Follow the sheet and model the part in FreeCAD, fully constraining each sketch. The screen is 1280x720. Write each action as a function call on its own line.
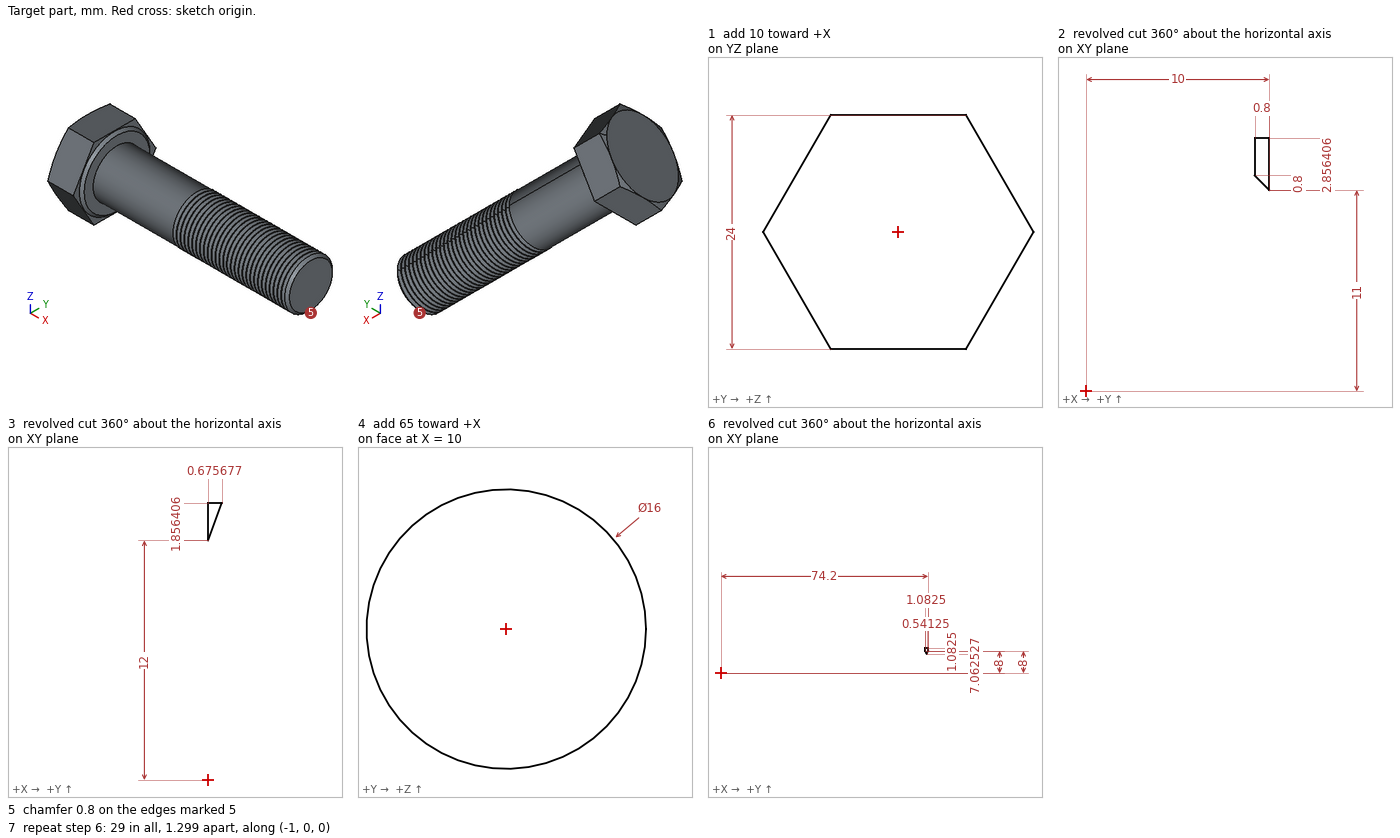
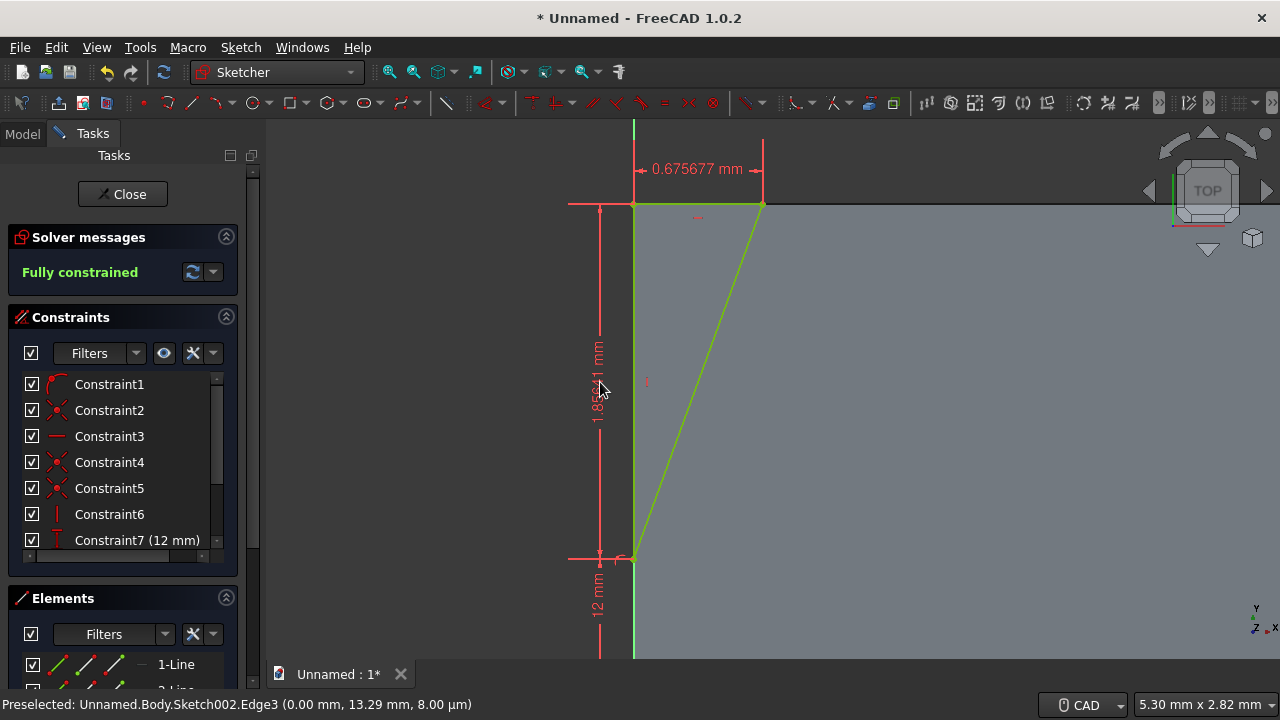
click(123, 194)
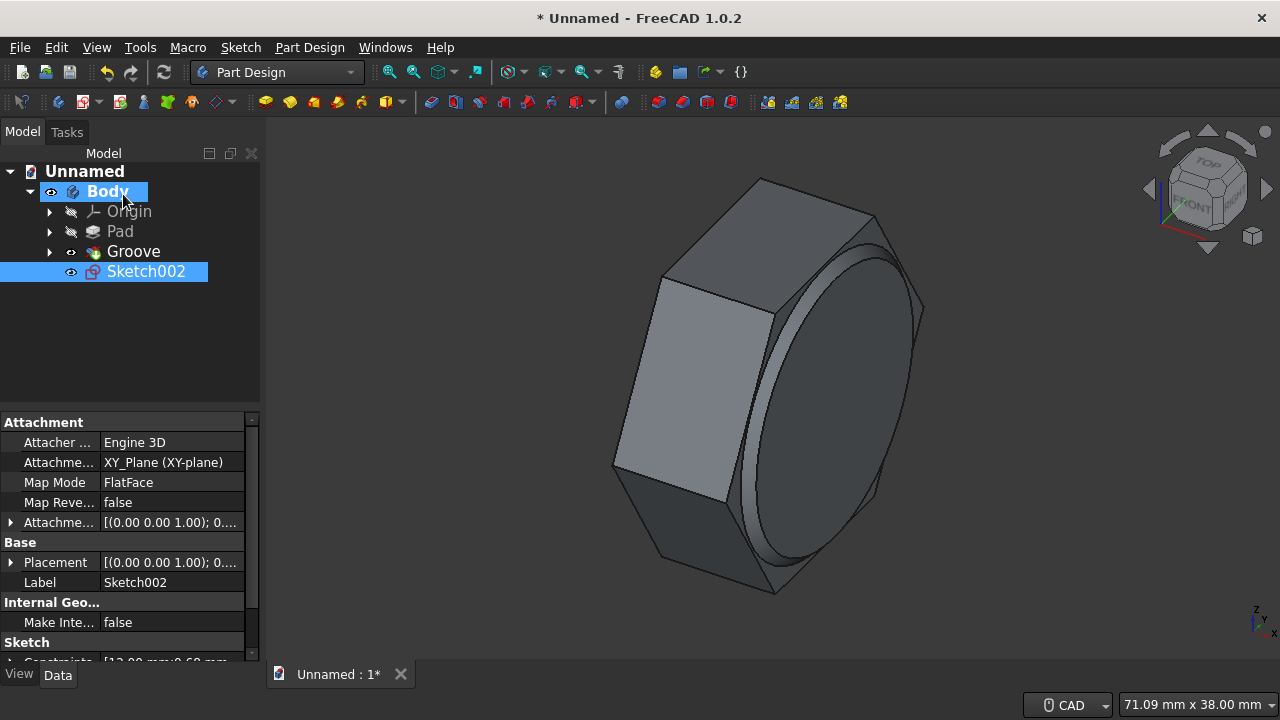
click(480, 102)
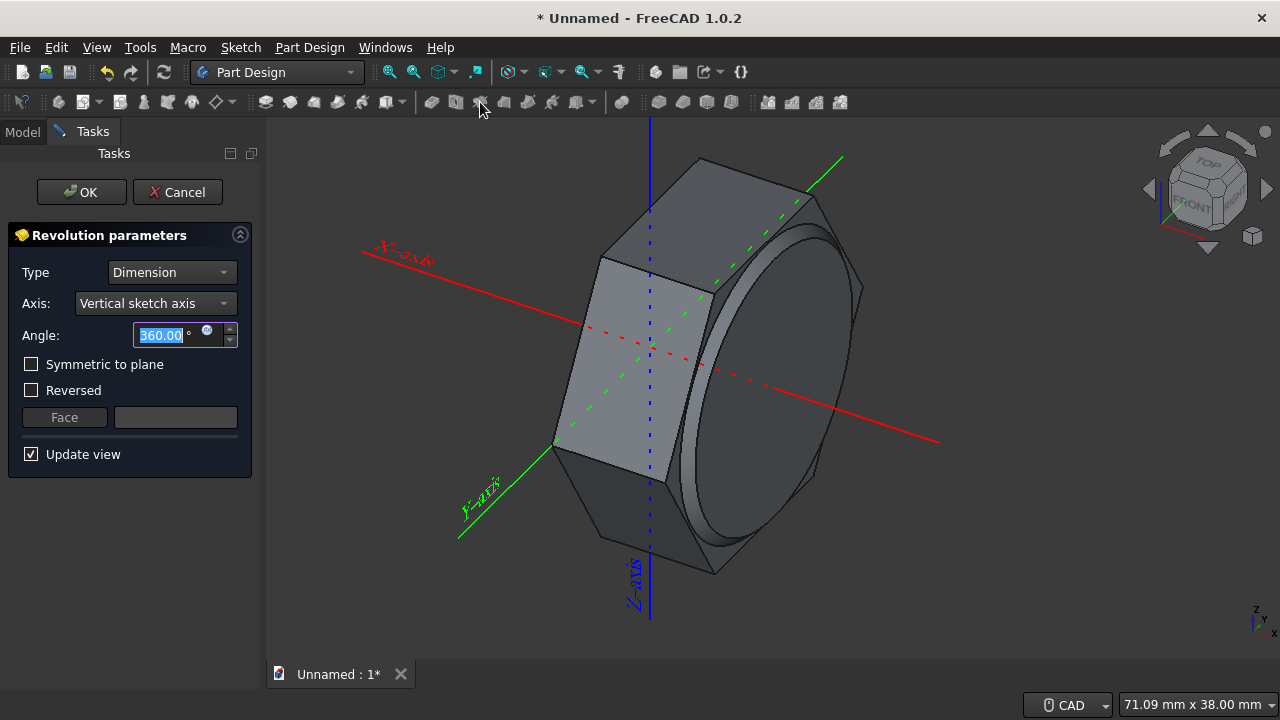
click(156, 304)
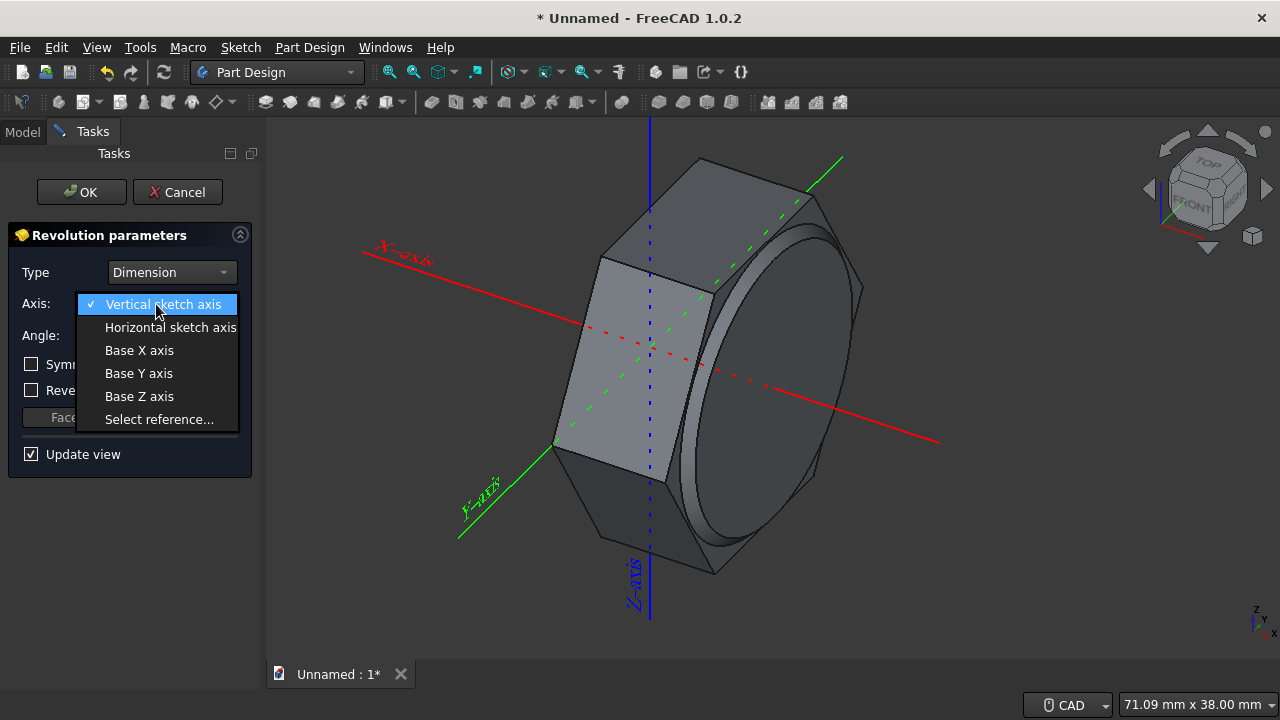
click(156, 328)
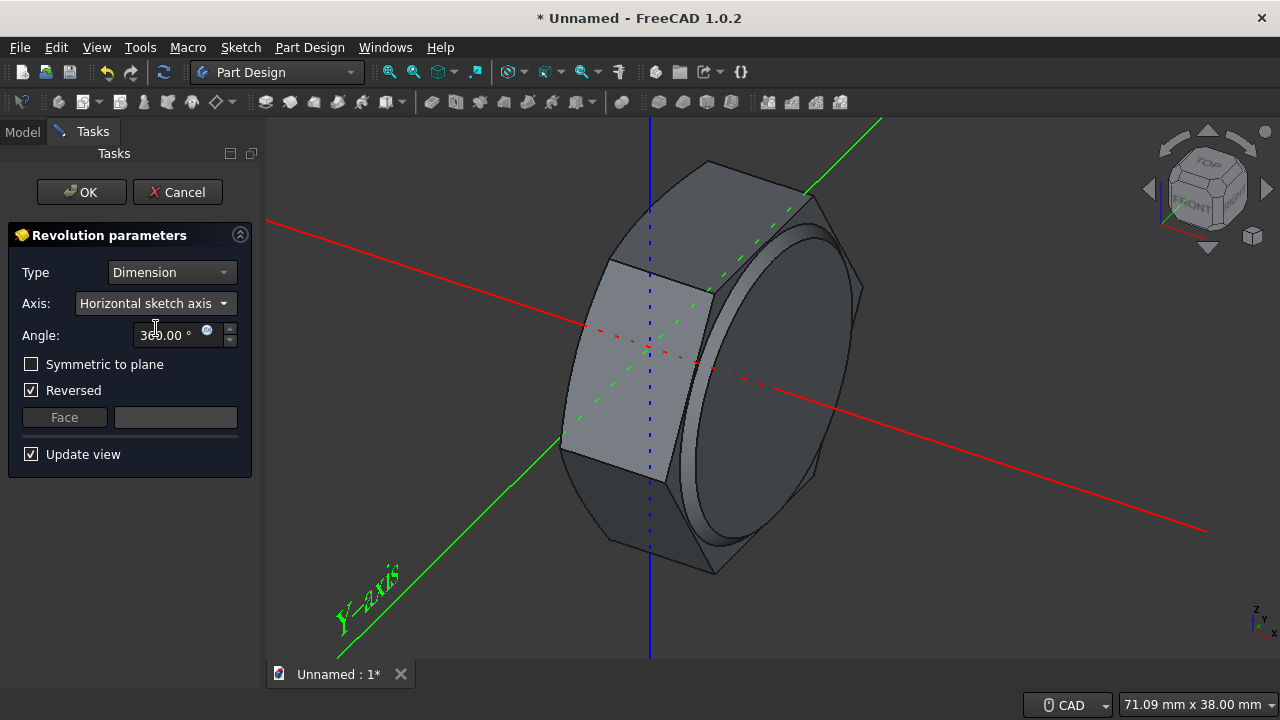
click(82, 192)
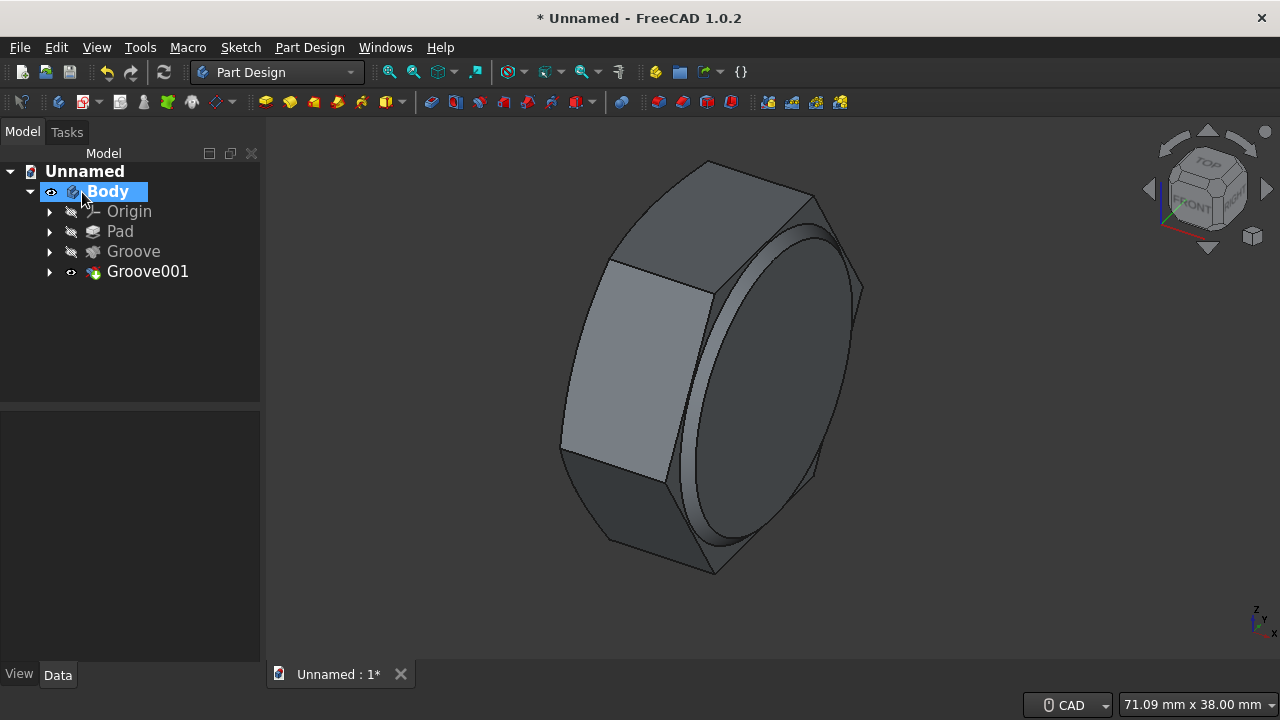
click(390, 72)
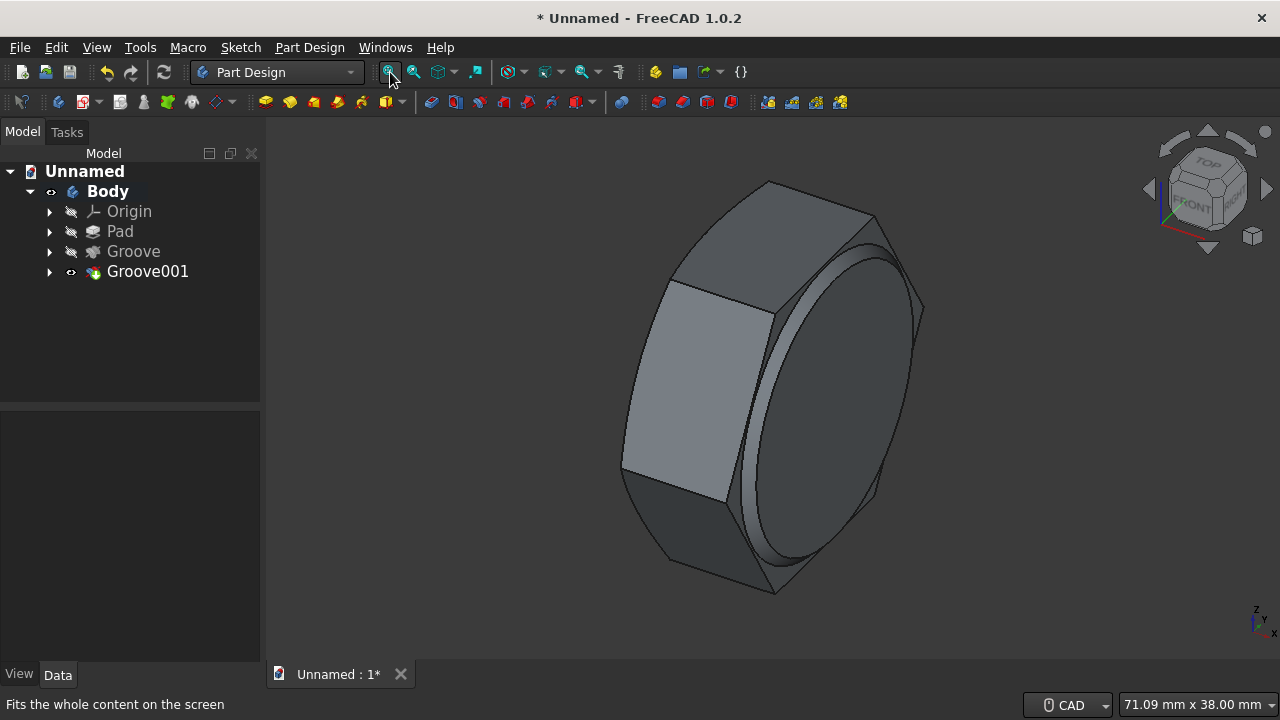
click(835, 407)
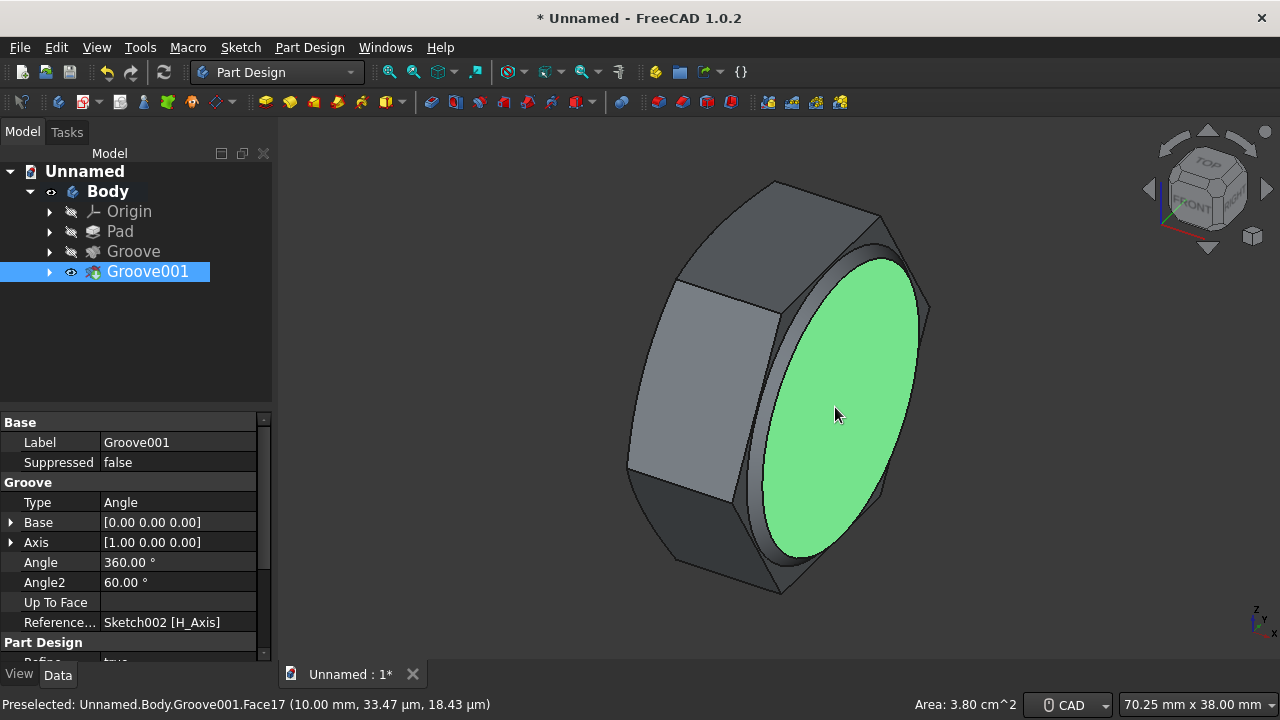
click(84, 102)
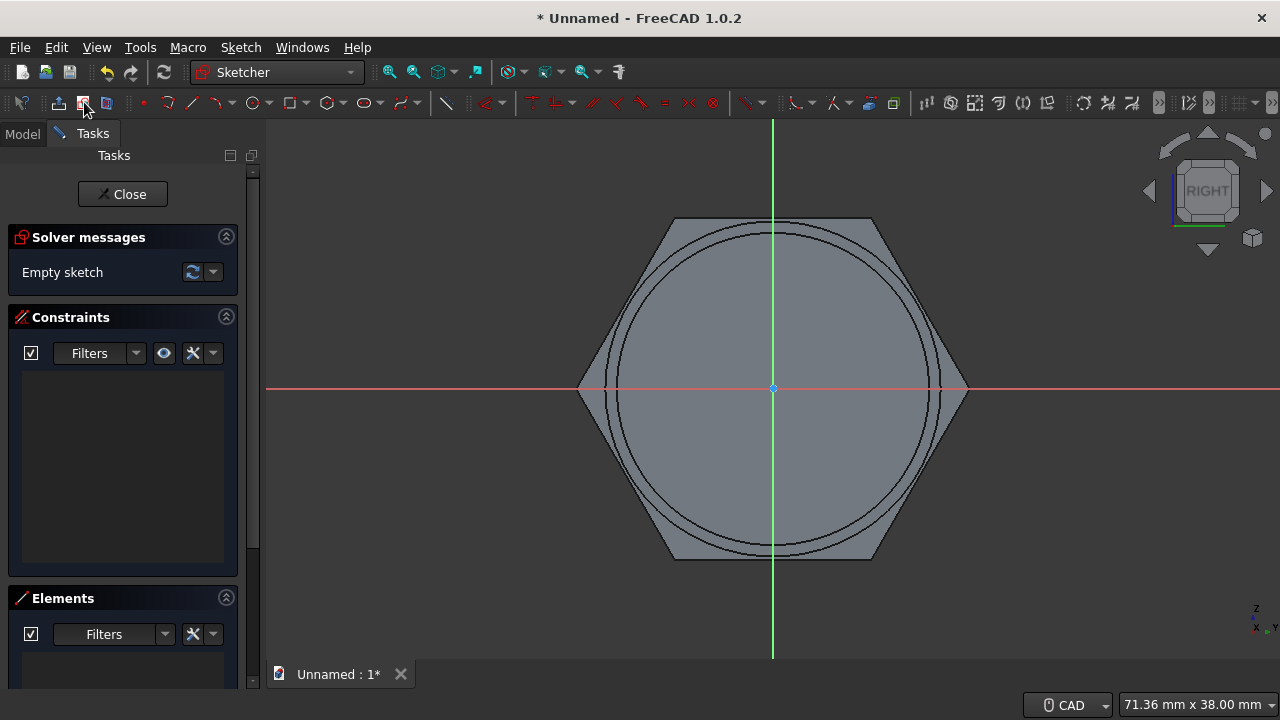
scroll(912, 389, up, 2)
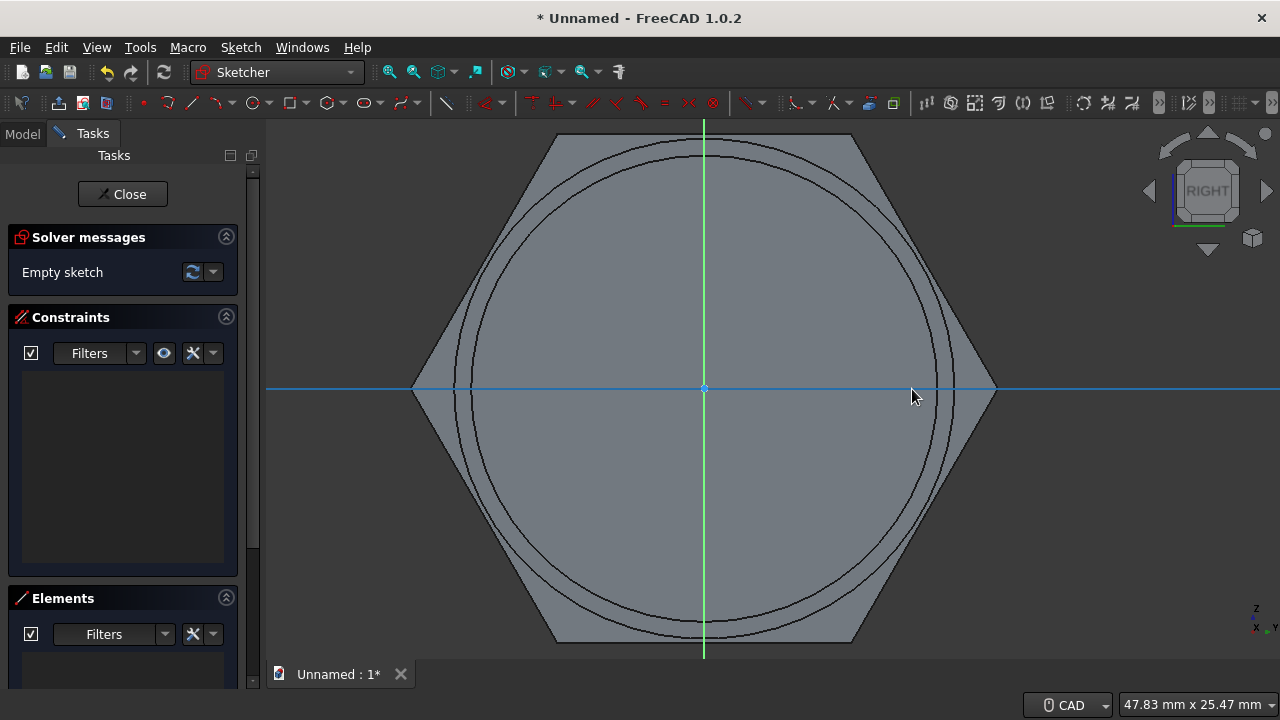
click(254, 104)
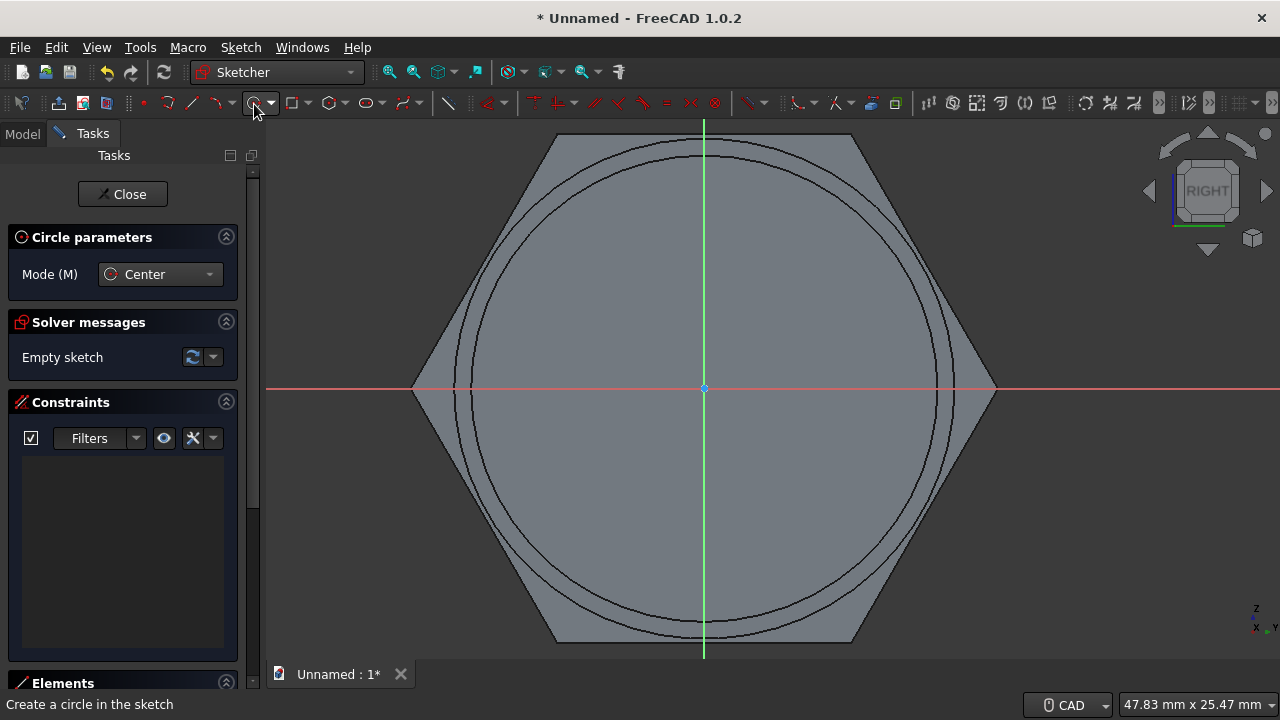
click(704, 389)
click(824, 269)
key(Escape)